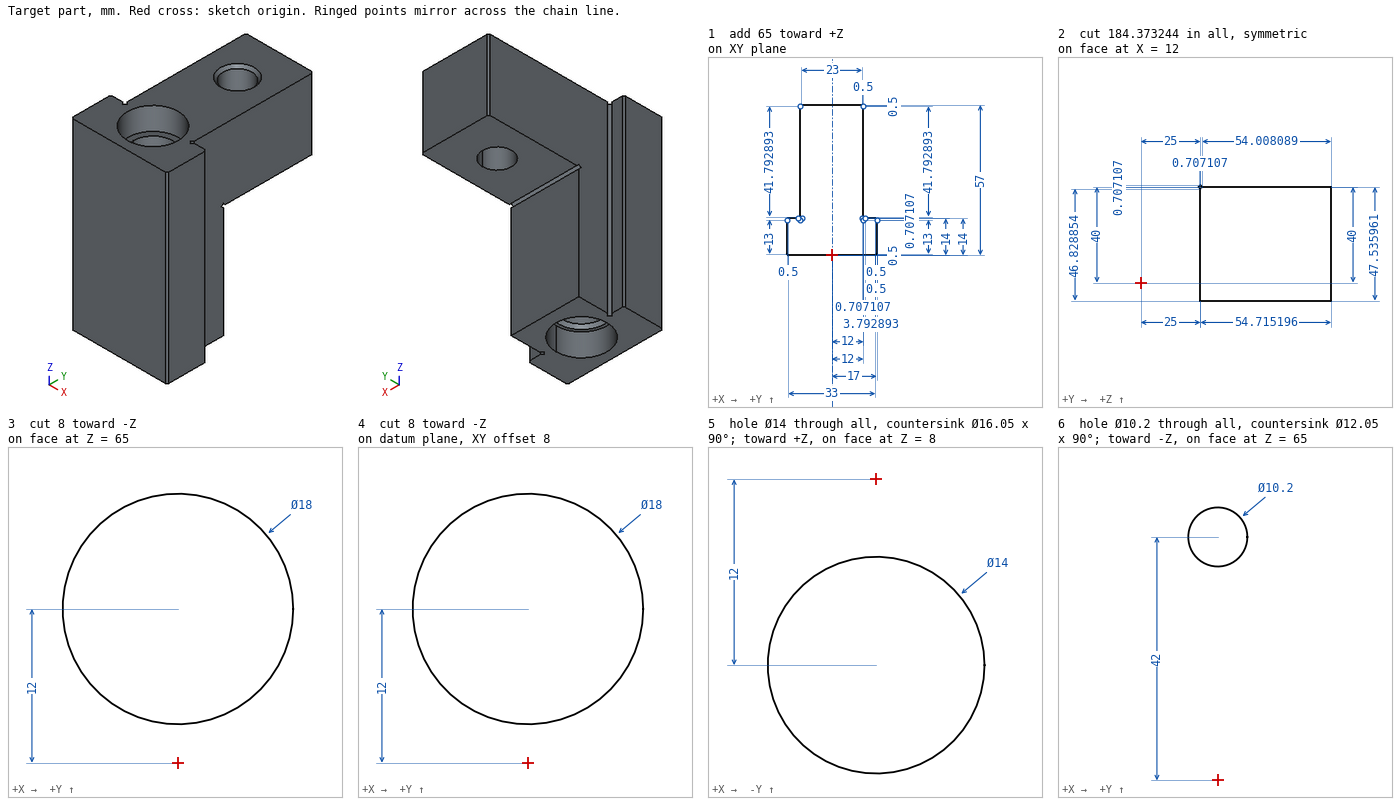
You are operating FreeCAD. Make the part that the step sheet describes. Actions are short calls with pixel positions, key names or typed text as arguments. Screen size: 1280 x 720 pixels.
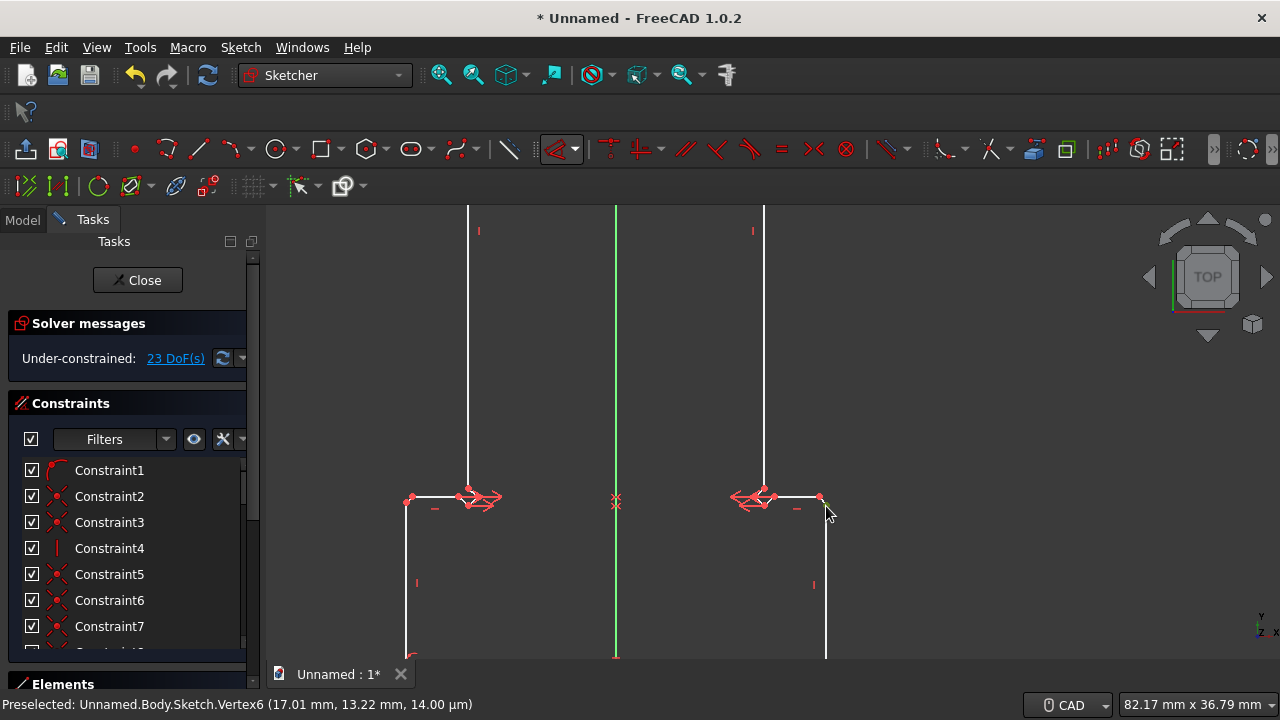
scroll(406, 503, up, 2)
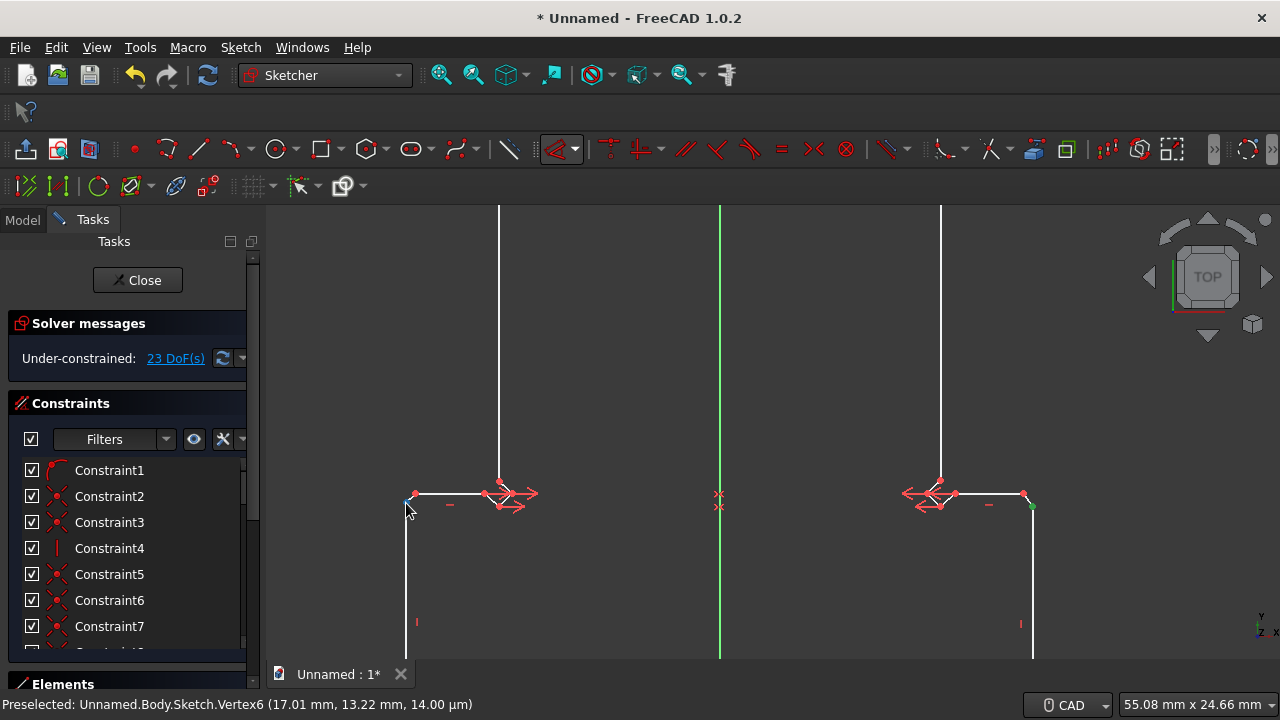
click(406, 502)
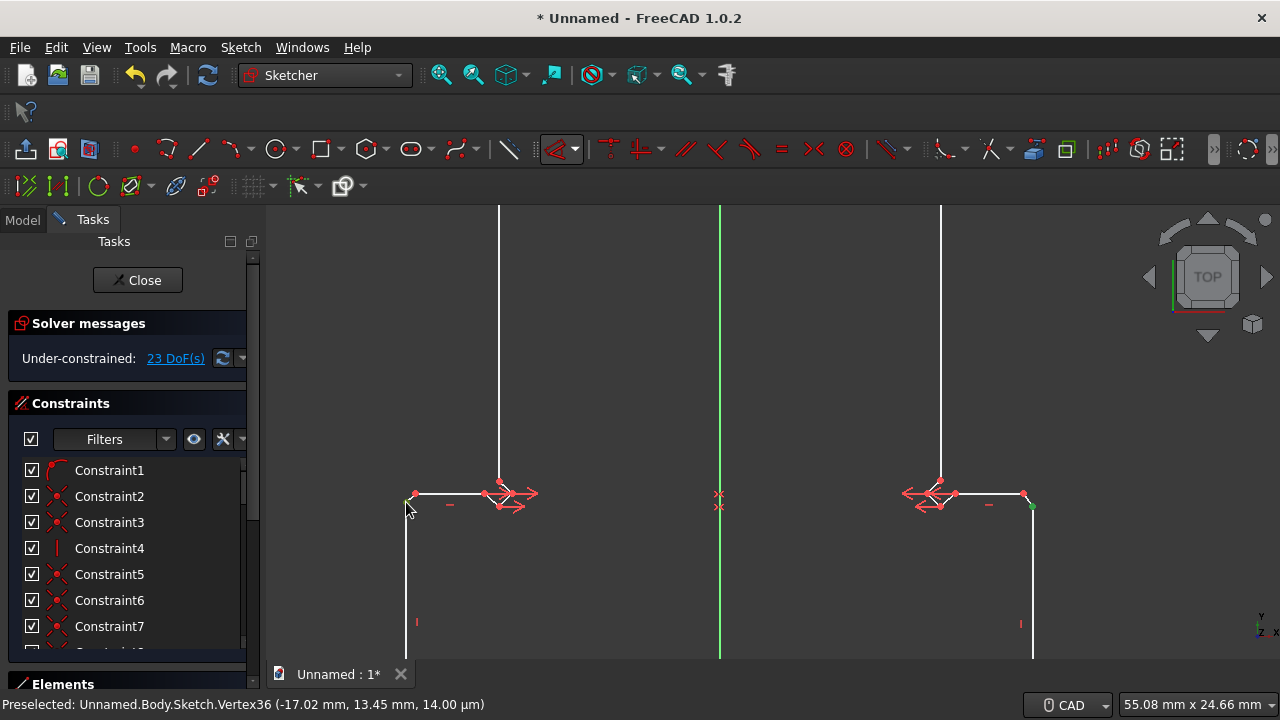
click(720, 603)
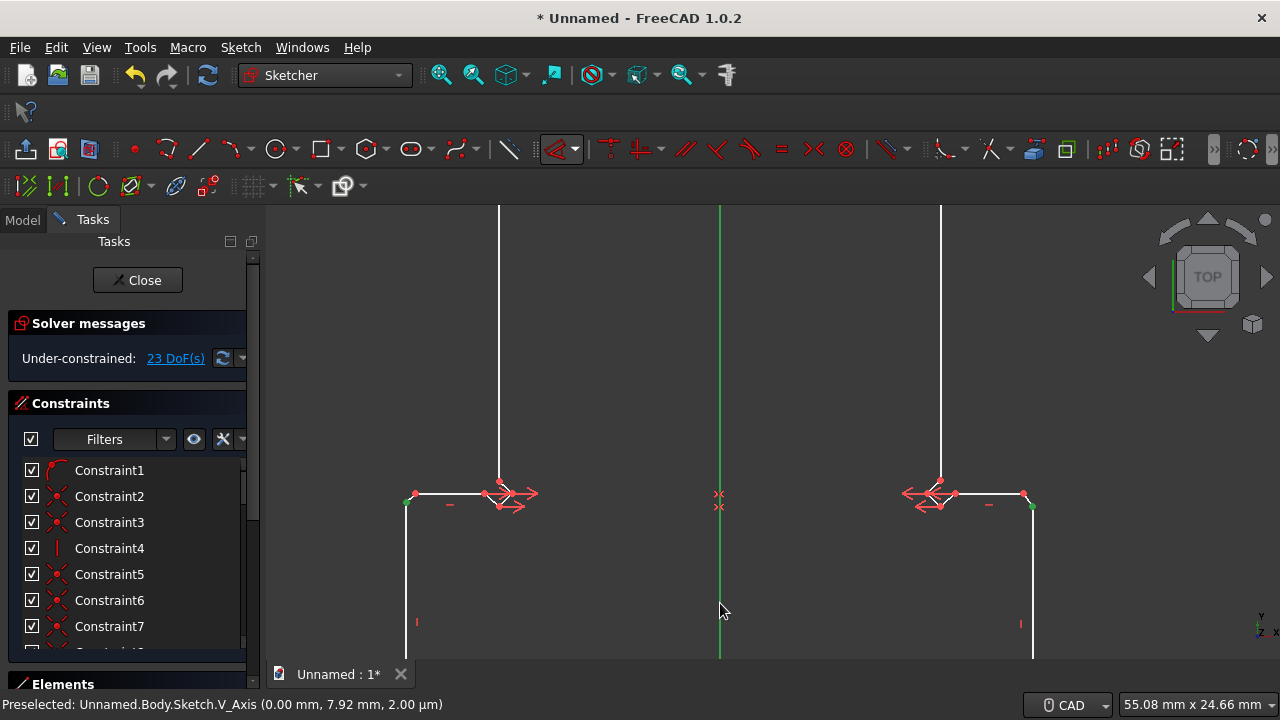
key(s)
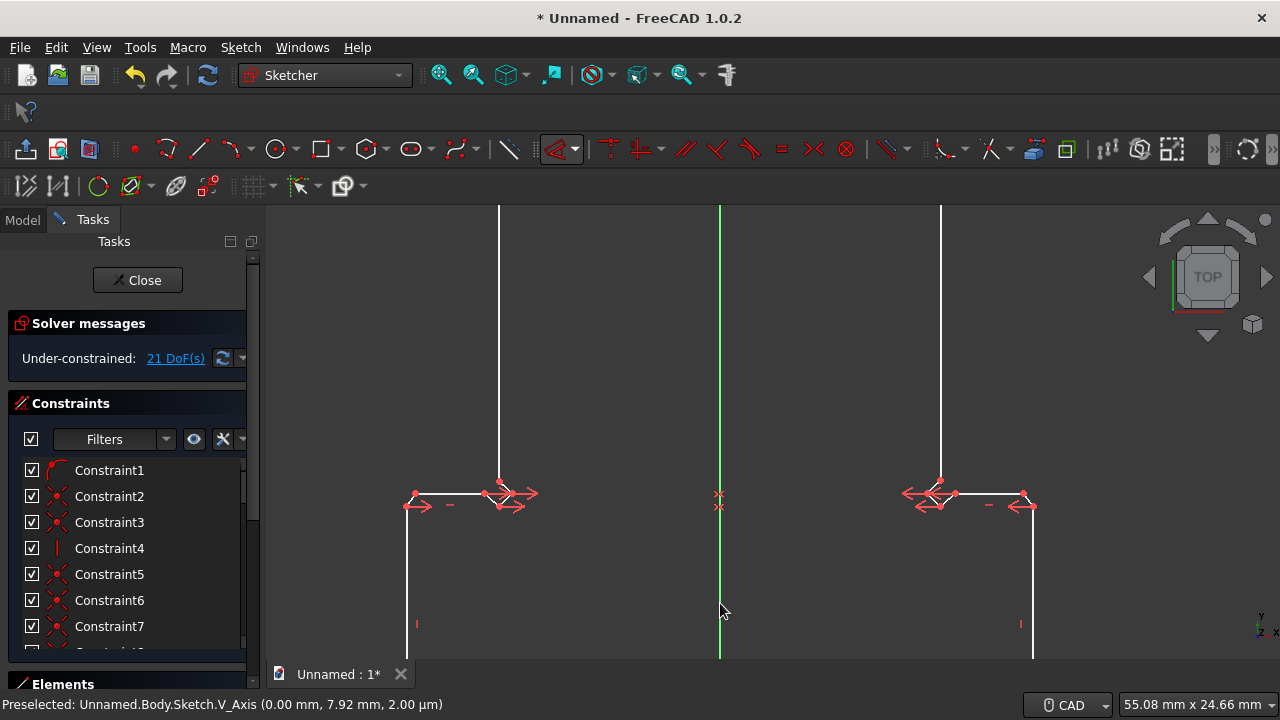
key(d)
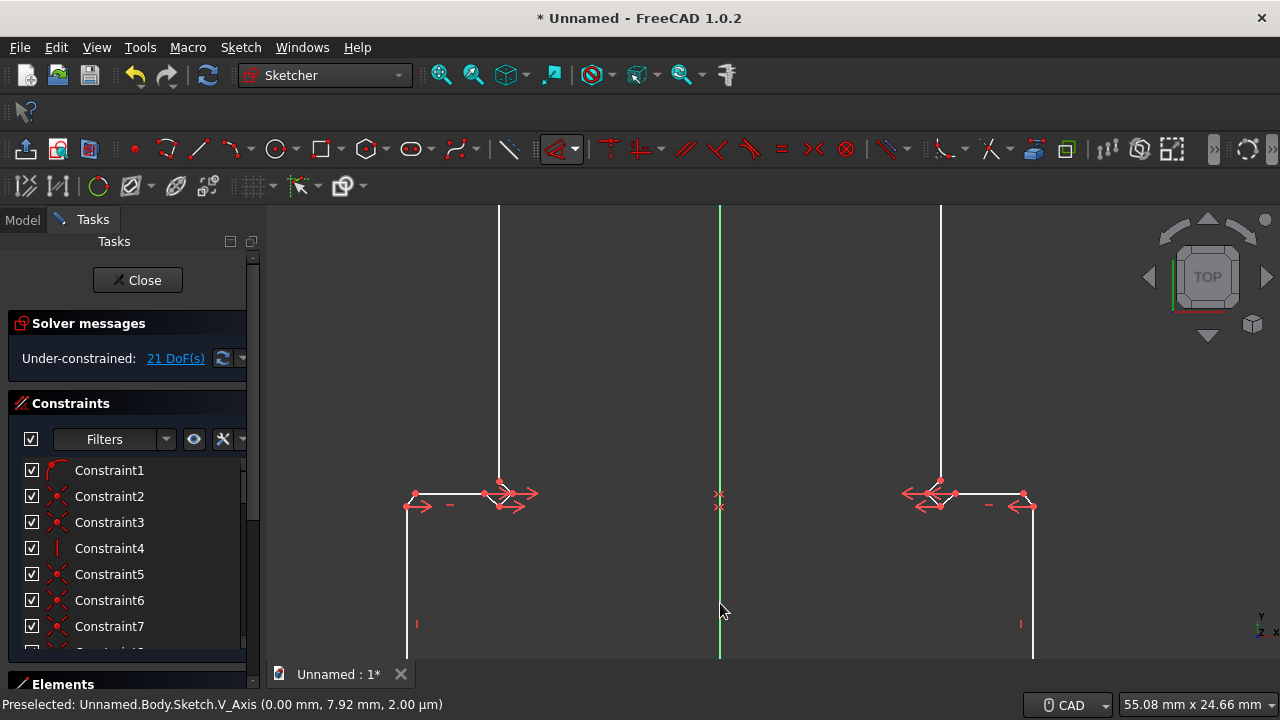
scroll(699, 500, down, 7)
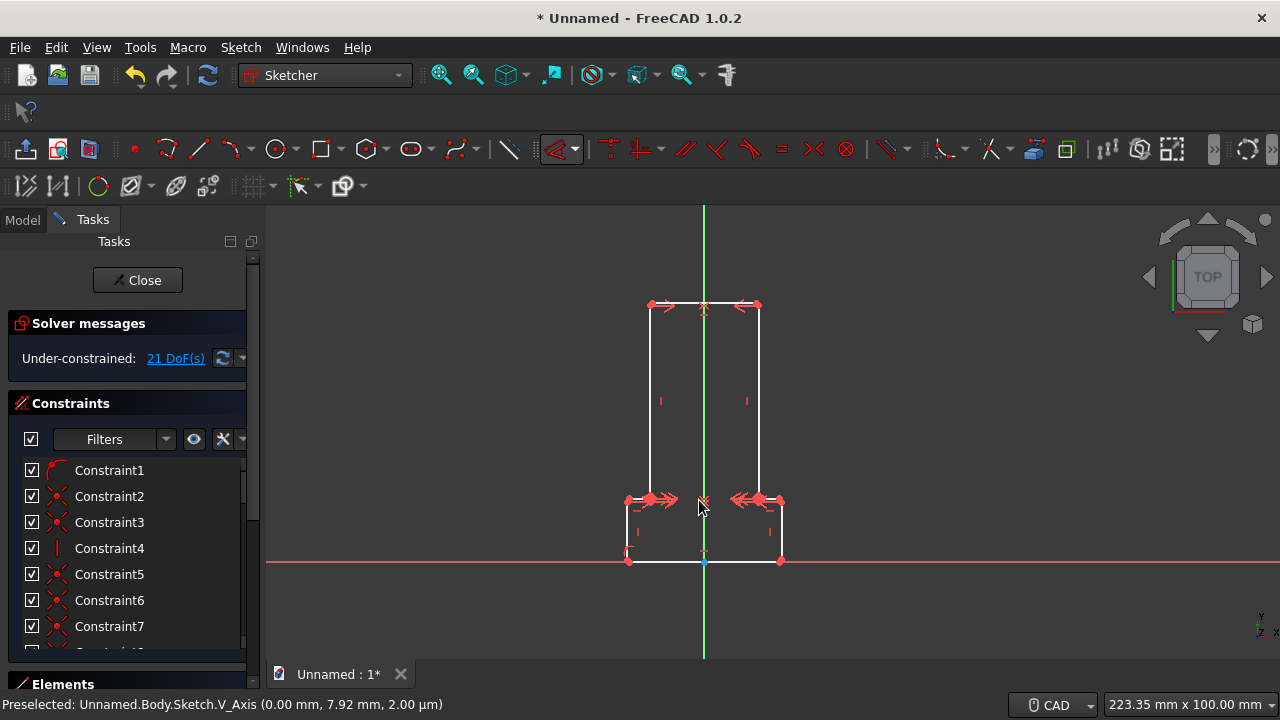
click(674, 562)
click(670, 596)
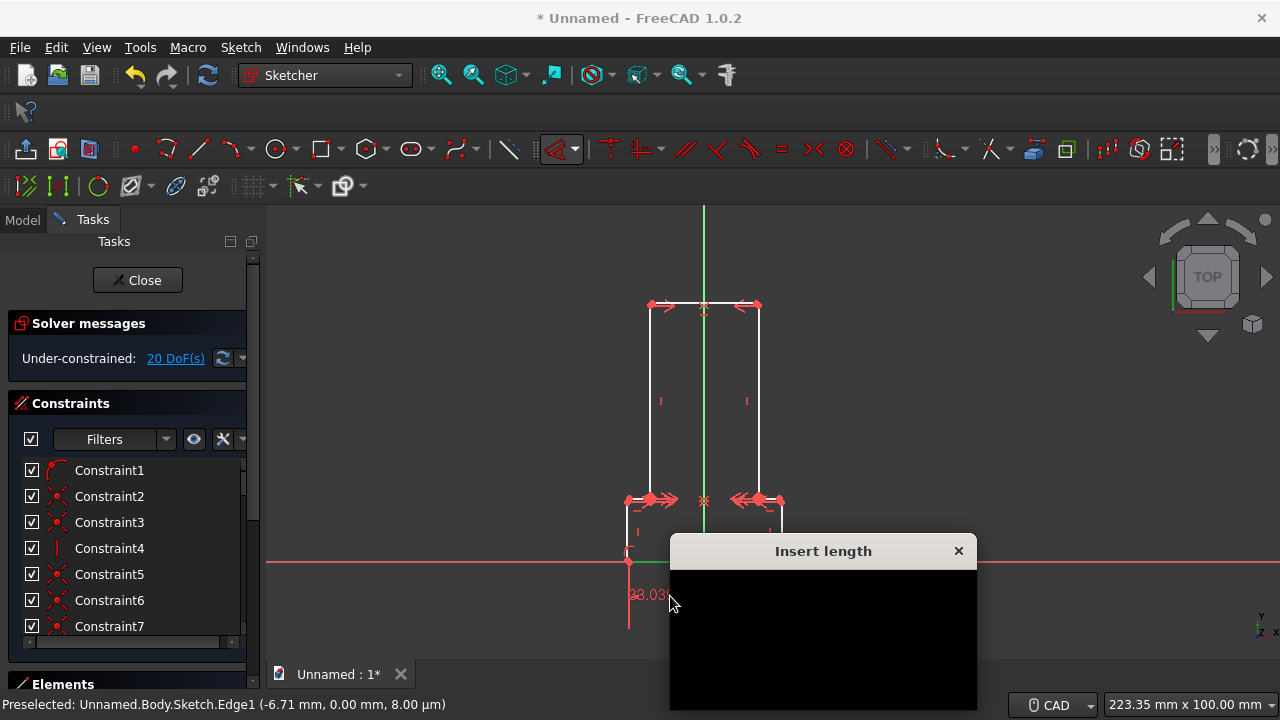
text(33)
key(Return)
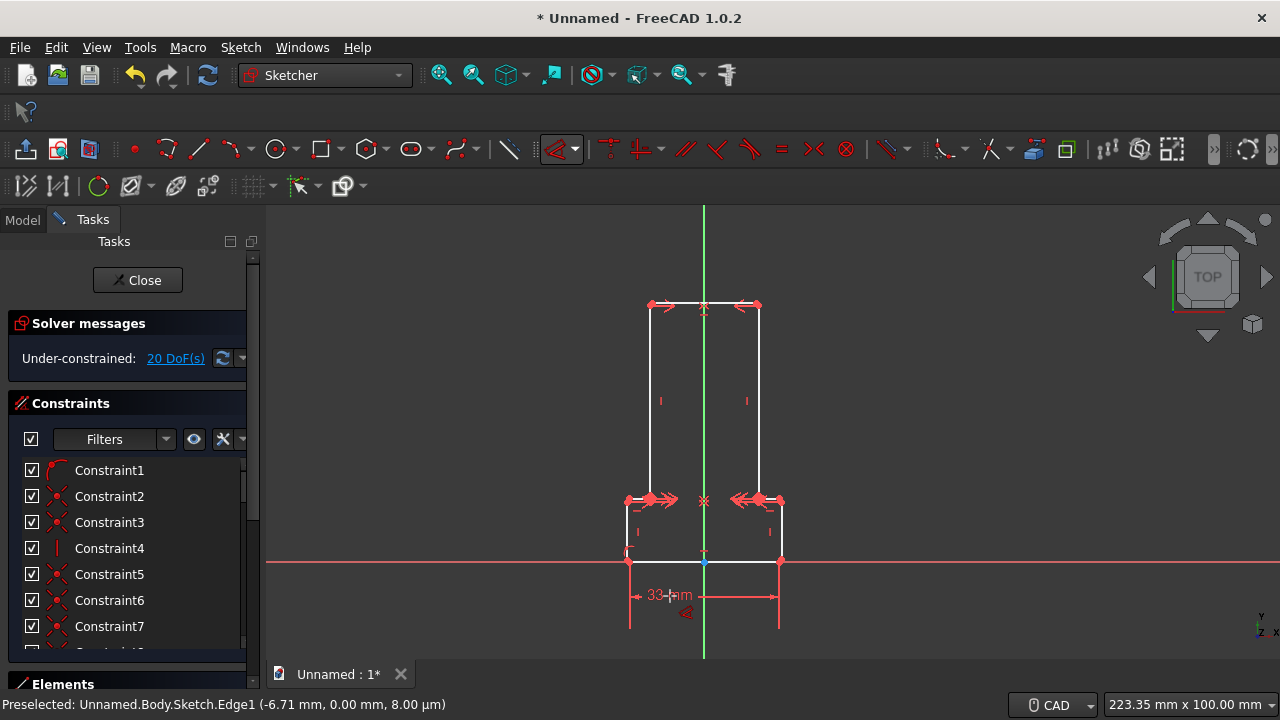
click(782, 543)
click(816, 531)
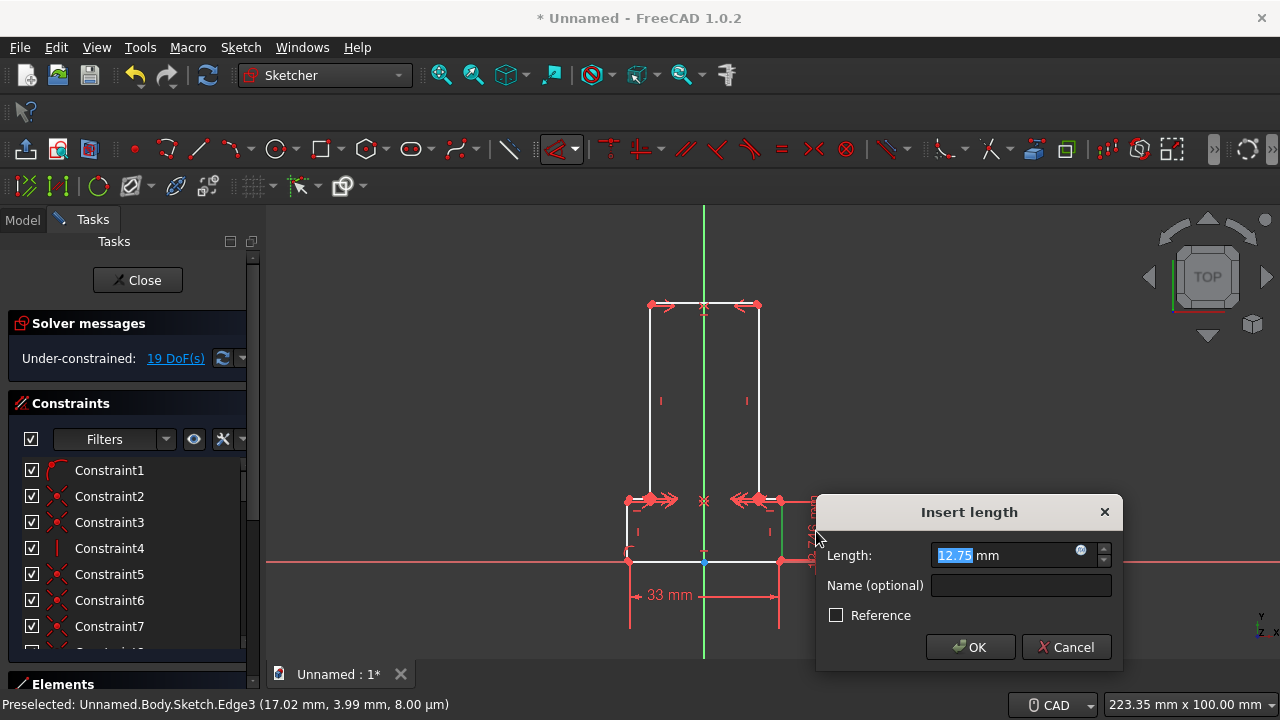
text(13)
key(Return)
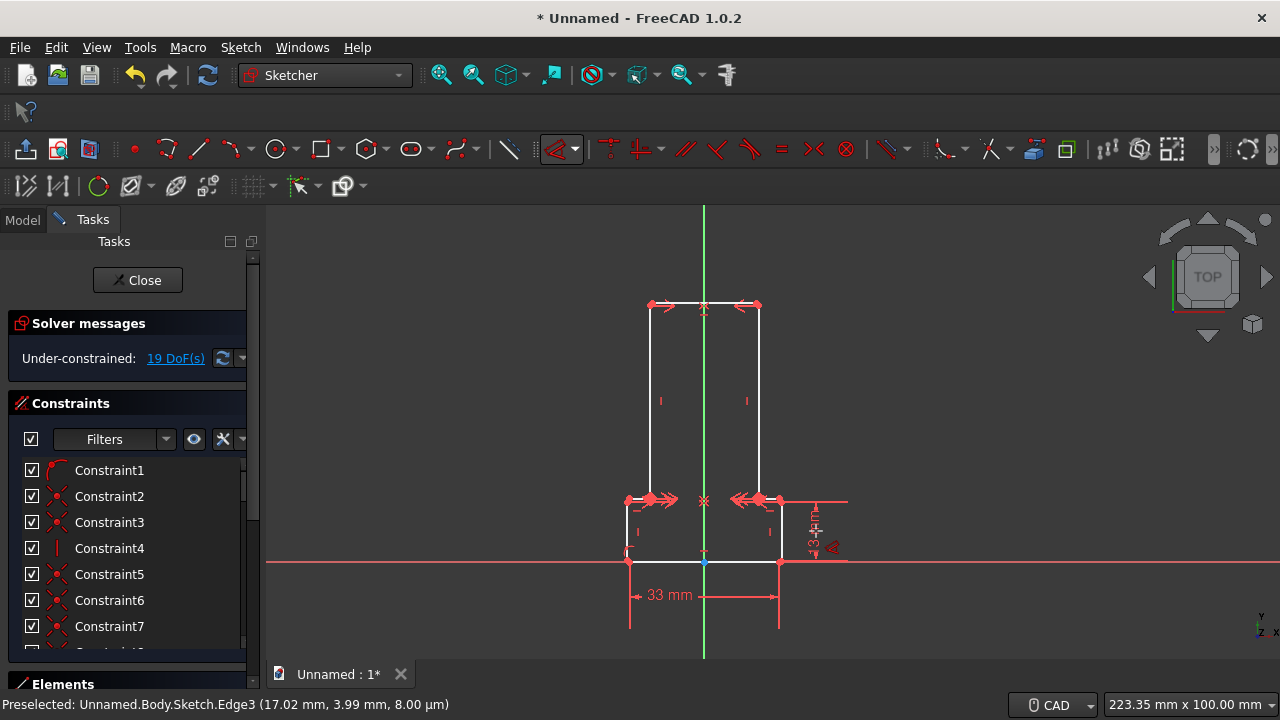
click(725, 303)
click(681, 269)